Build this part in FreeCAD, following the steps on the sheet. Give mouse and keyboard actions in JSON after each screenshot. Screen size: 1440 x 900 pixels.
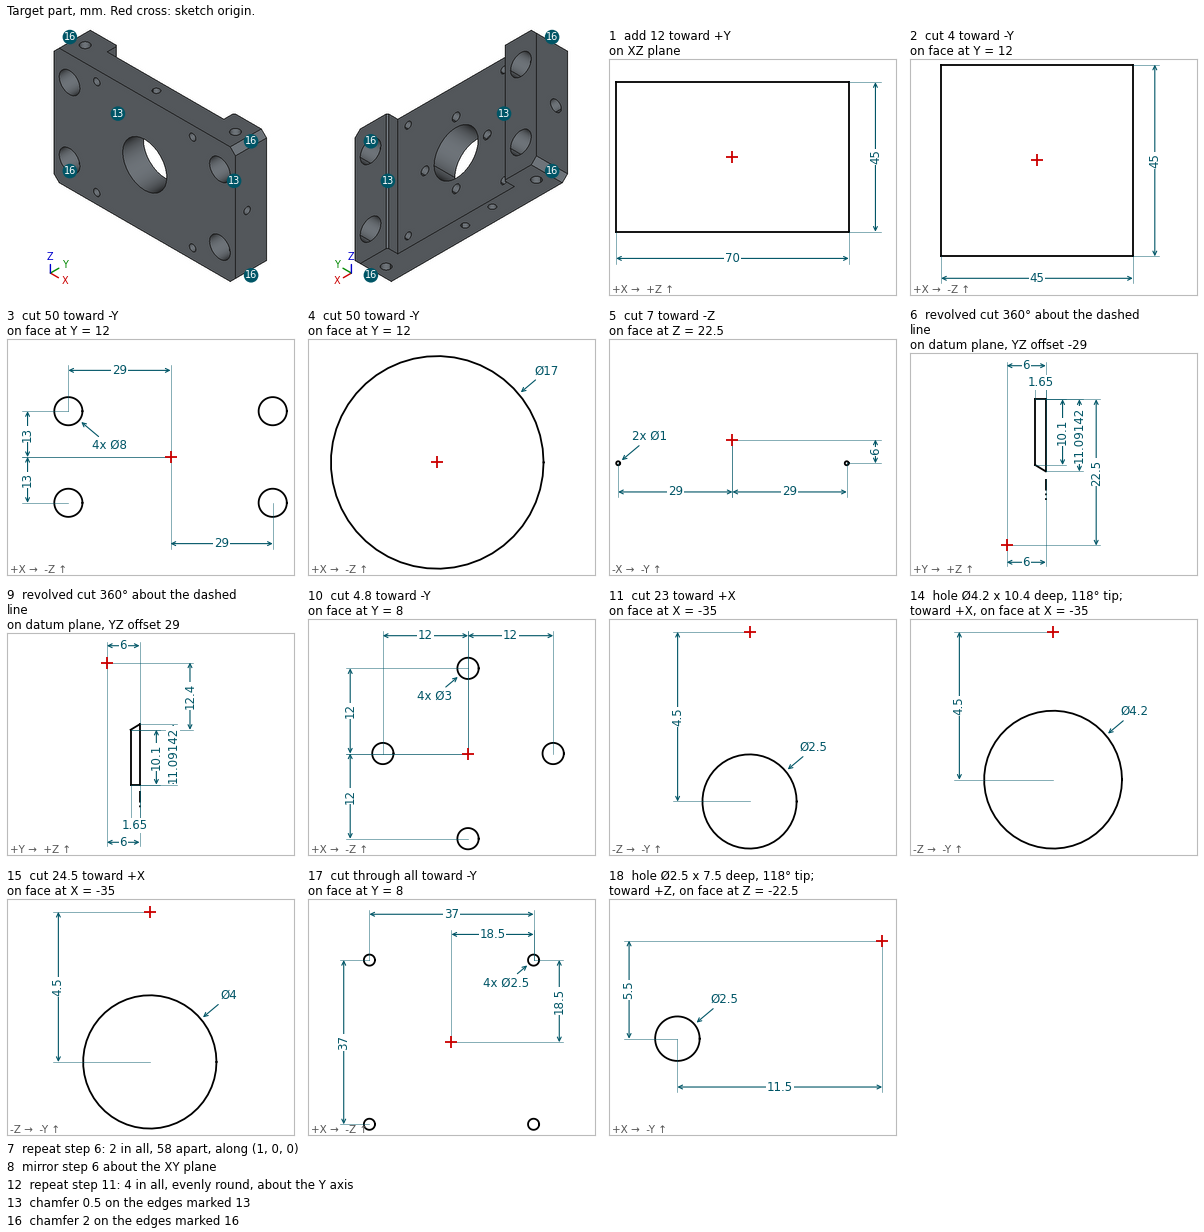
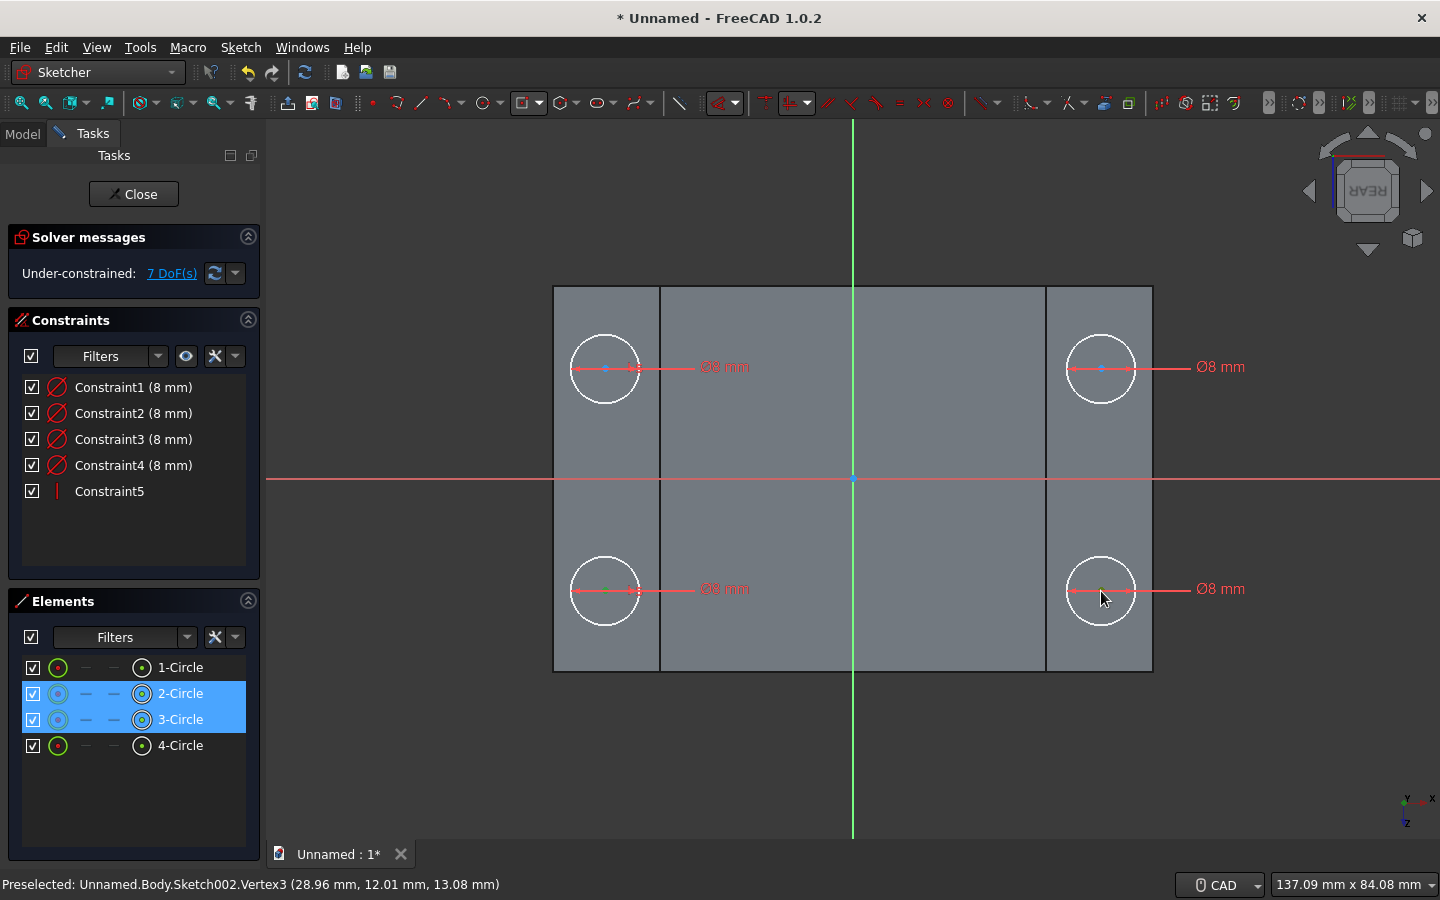
{"action": "left_click", "coordinate": [810, 104]}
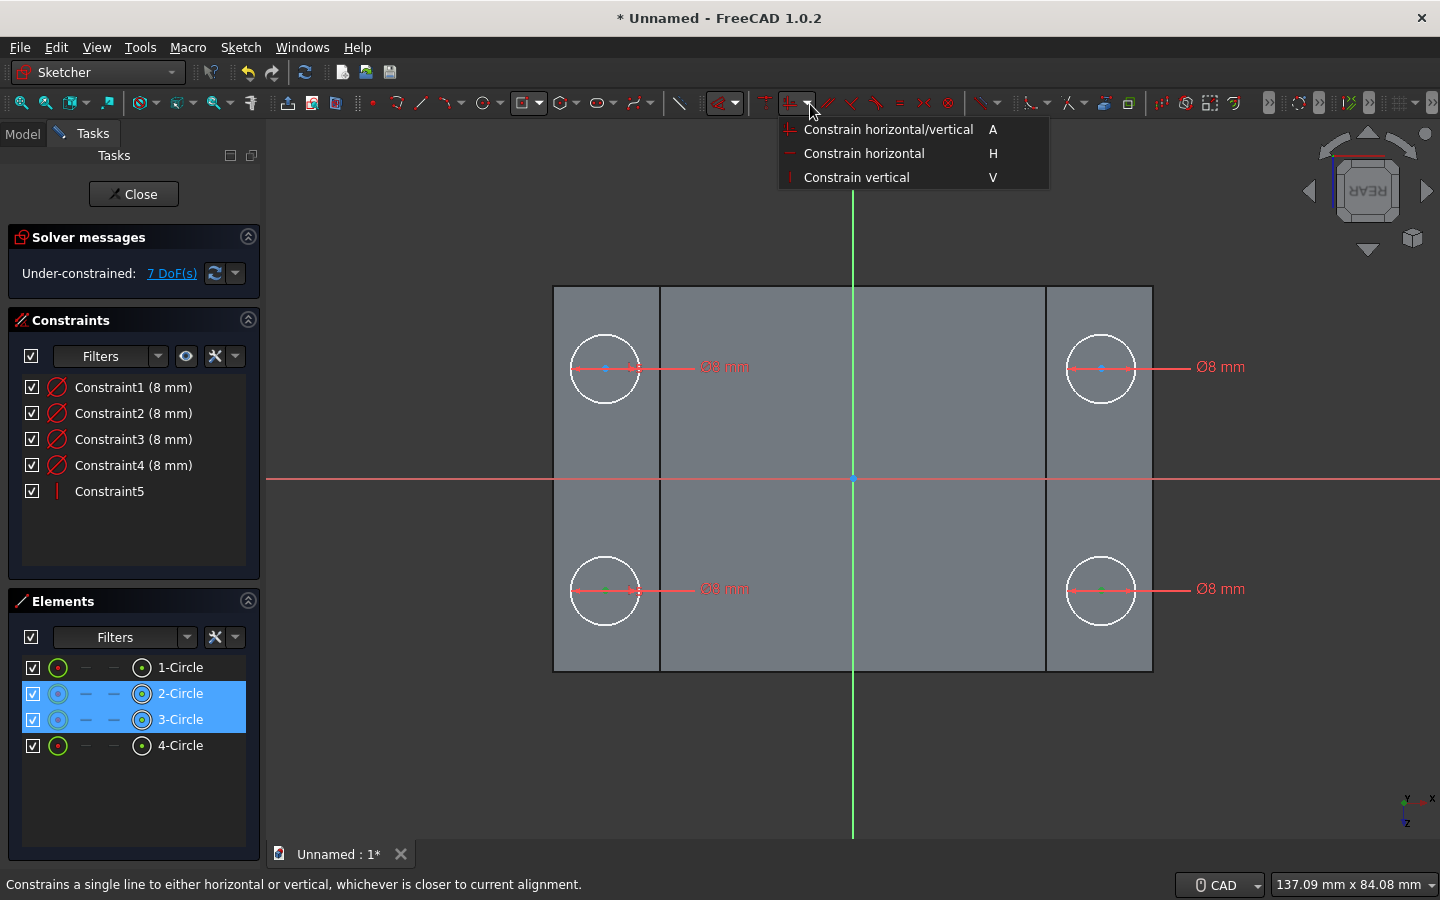
{"action": "left_click", "coordinate": [914, 153]}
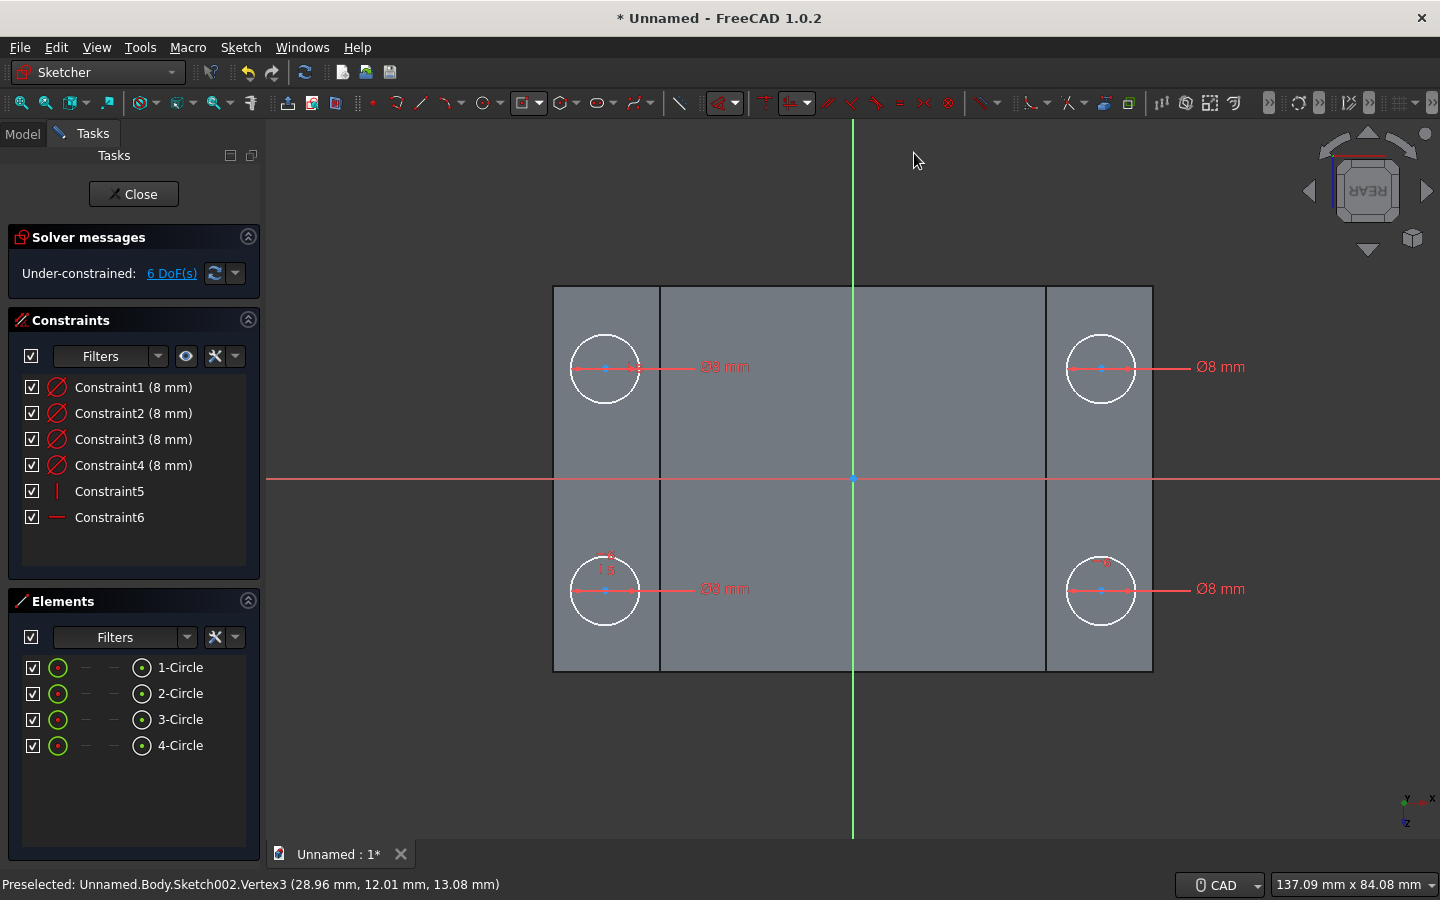
{"action": "left_click", "coordinate": [1101, 591]}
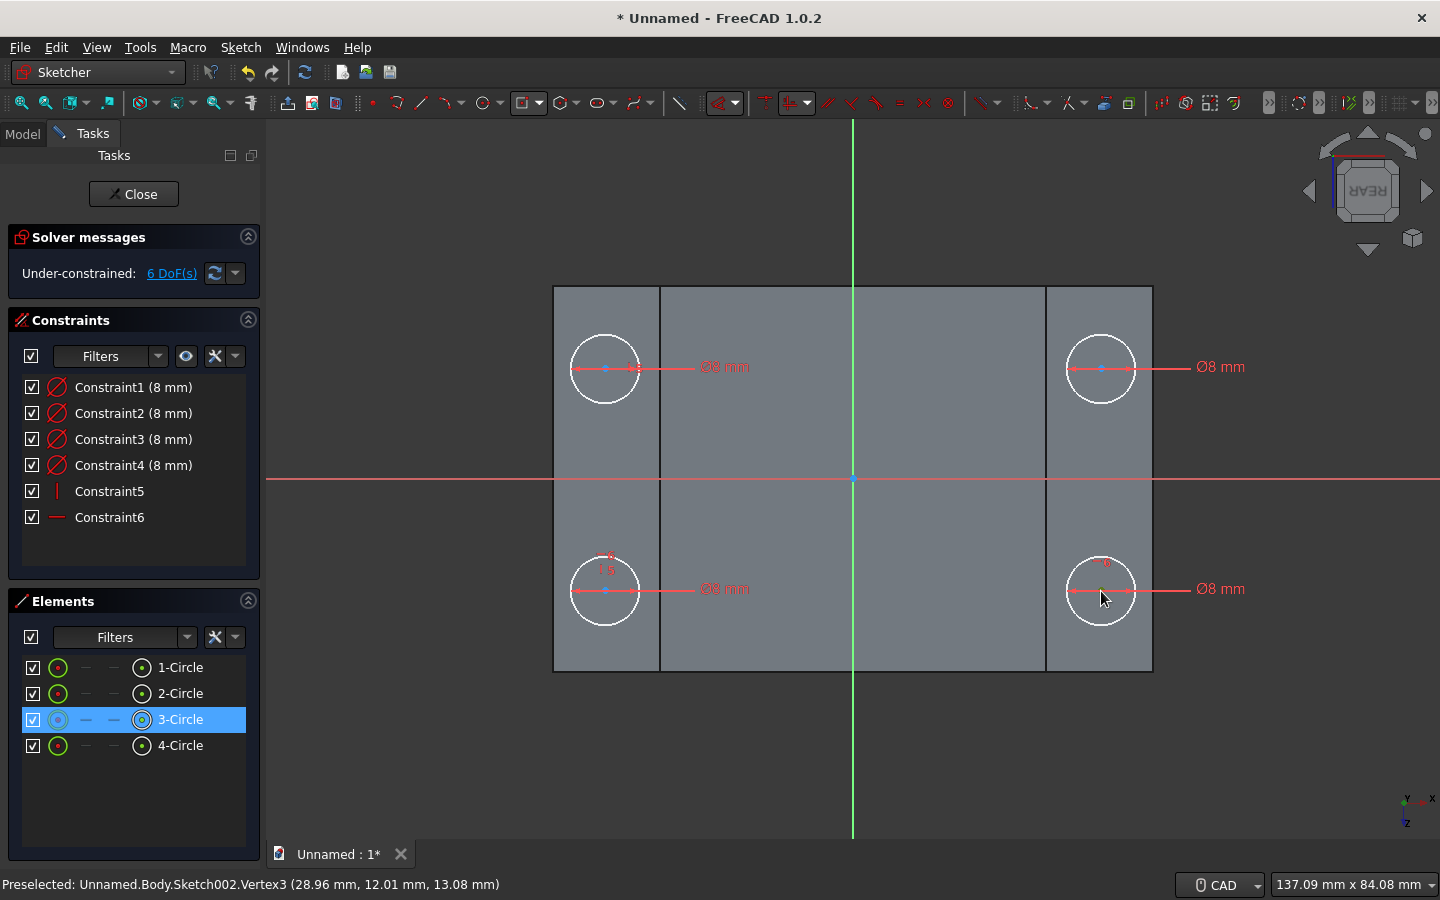
{"action": "left_click", "coordinate": [1101, 369]}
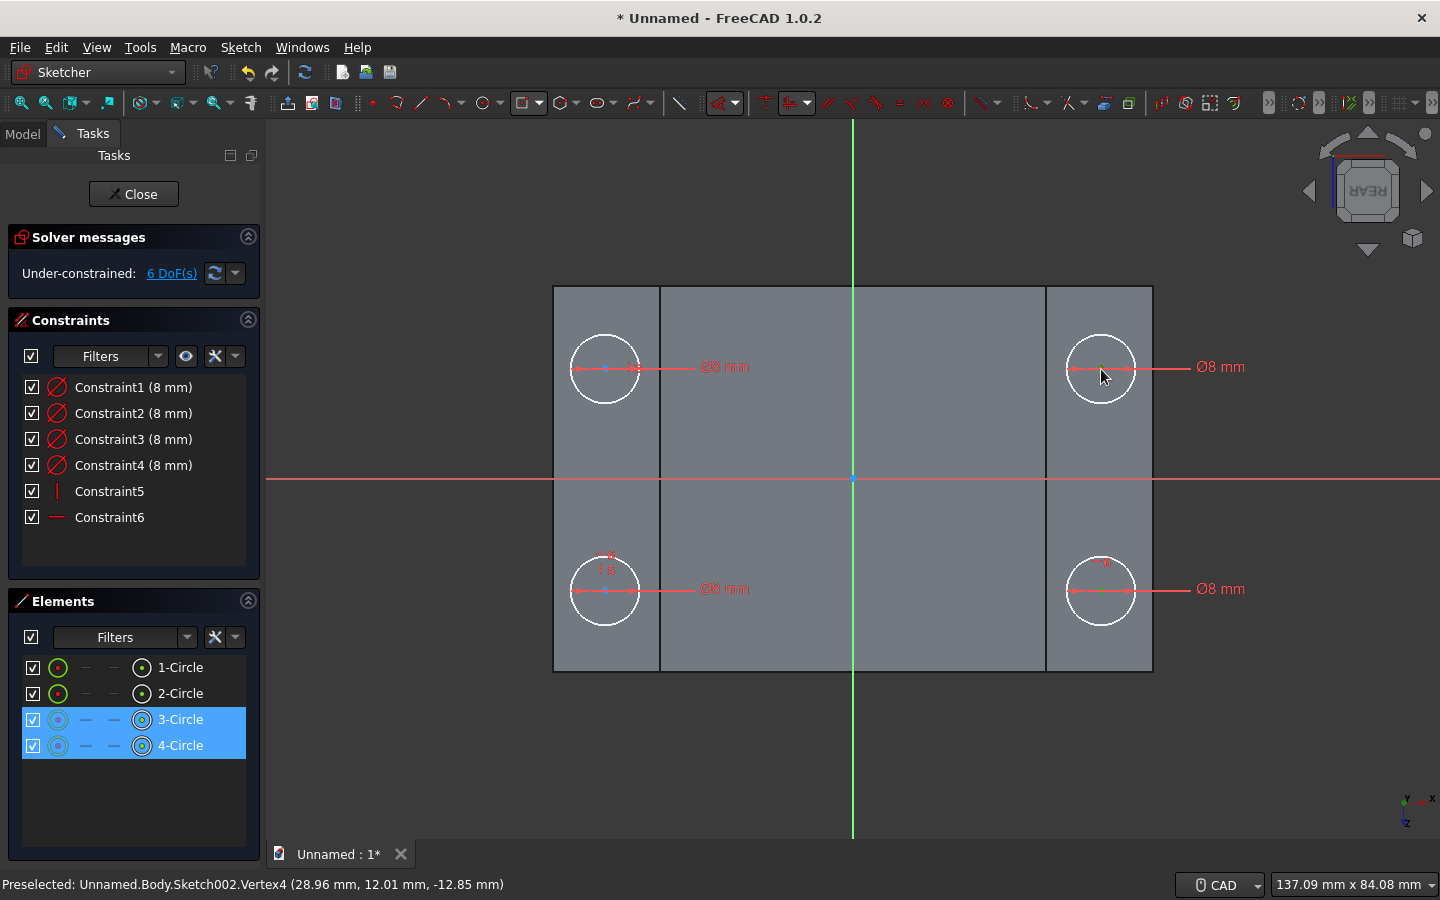
{"action": "key", "text": "v"}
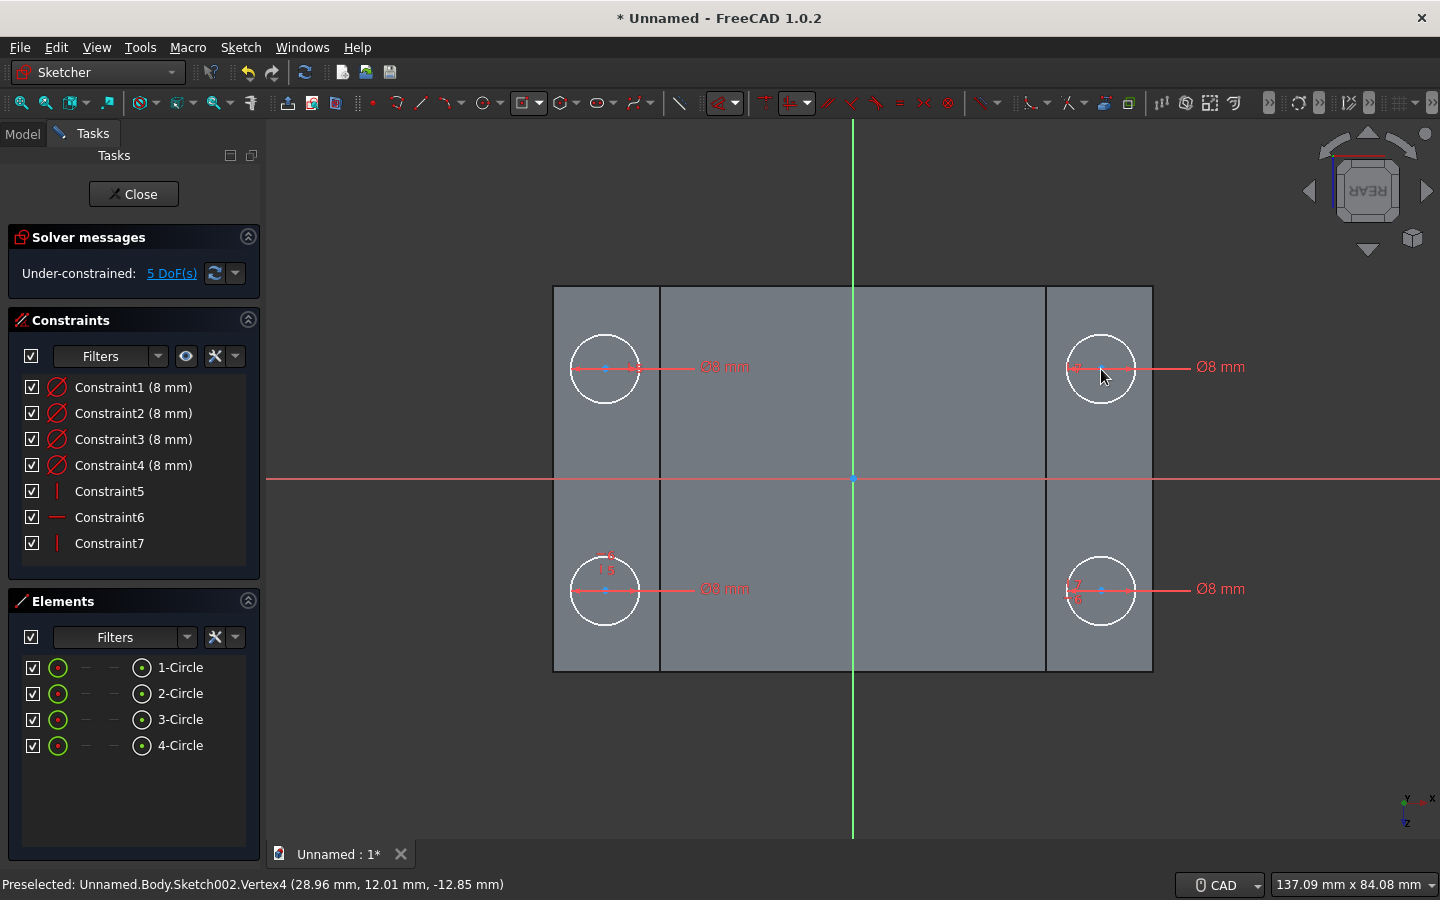
{"action": "left_click", "coordinate": [605, 369]}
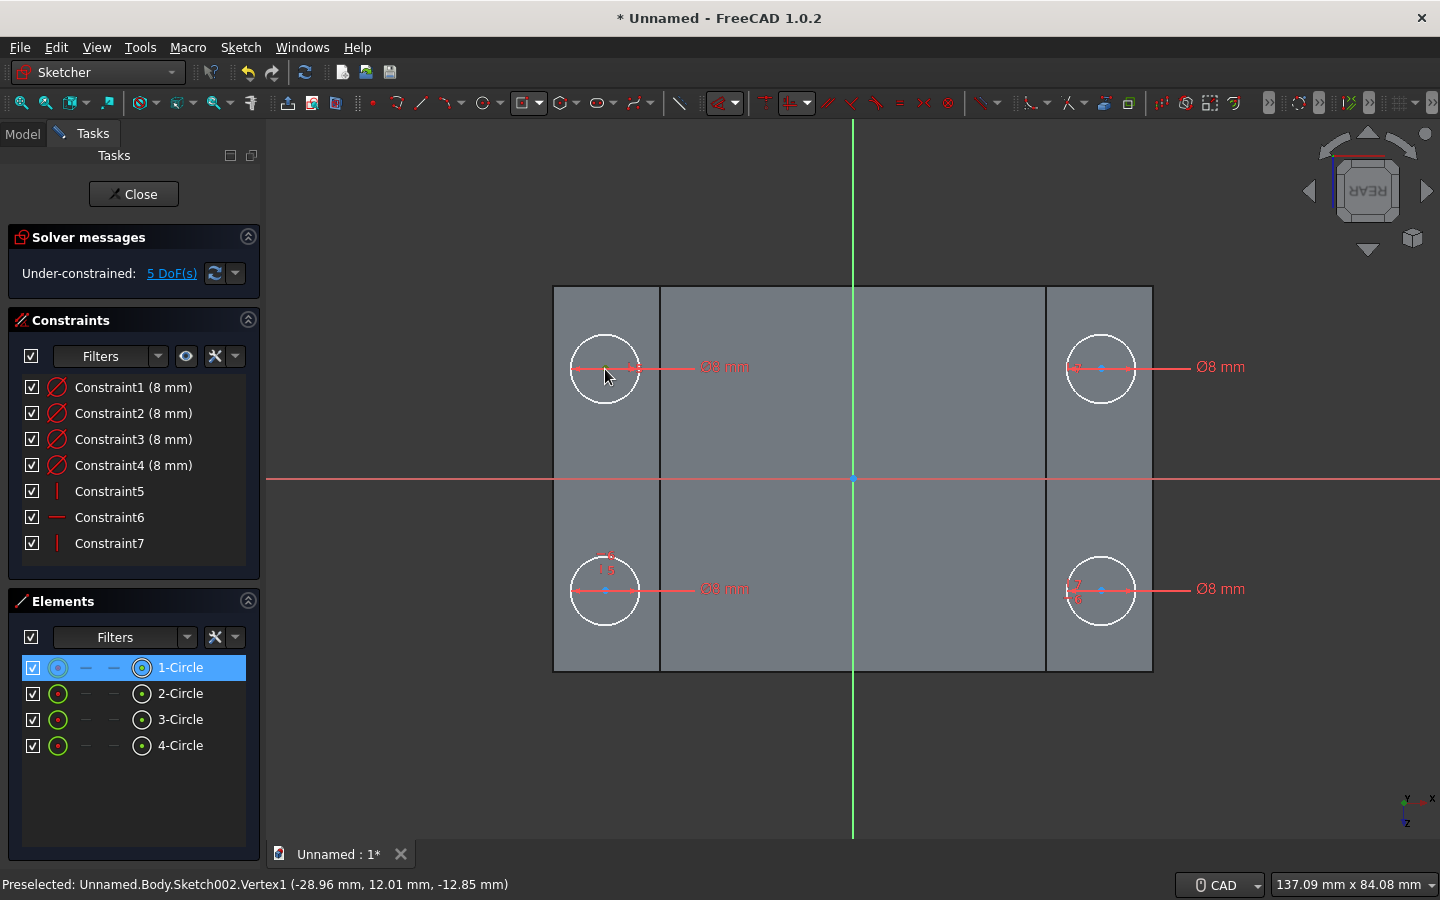
{"action": "left_click", "coordinate": [1101, 369]}